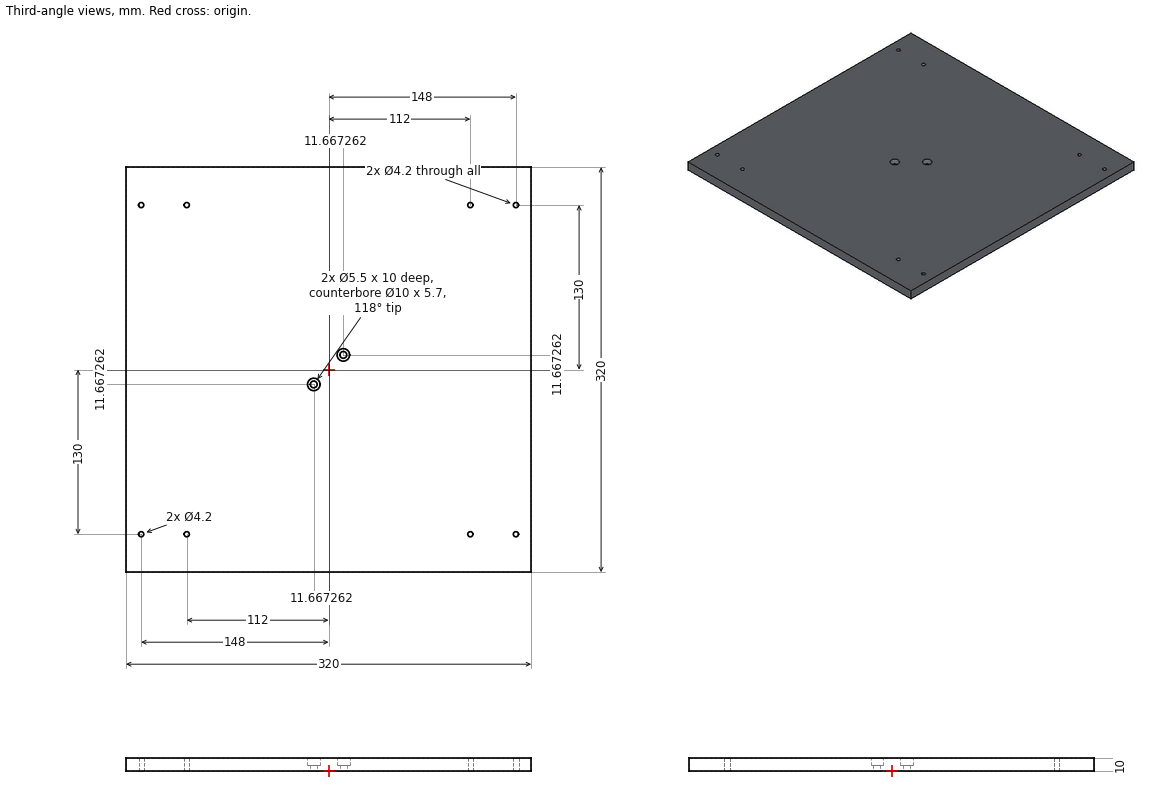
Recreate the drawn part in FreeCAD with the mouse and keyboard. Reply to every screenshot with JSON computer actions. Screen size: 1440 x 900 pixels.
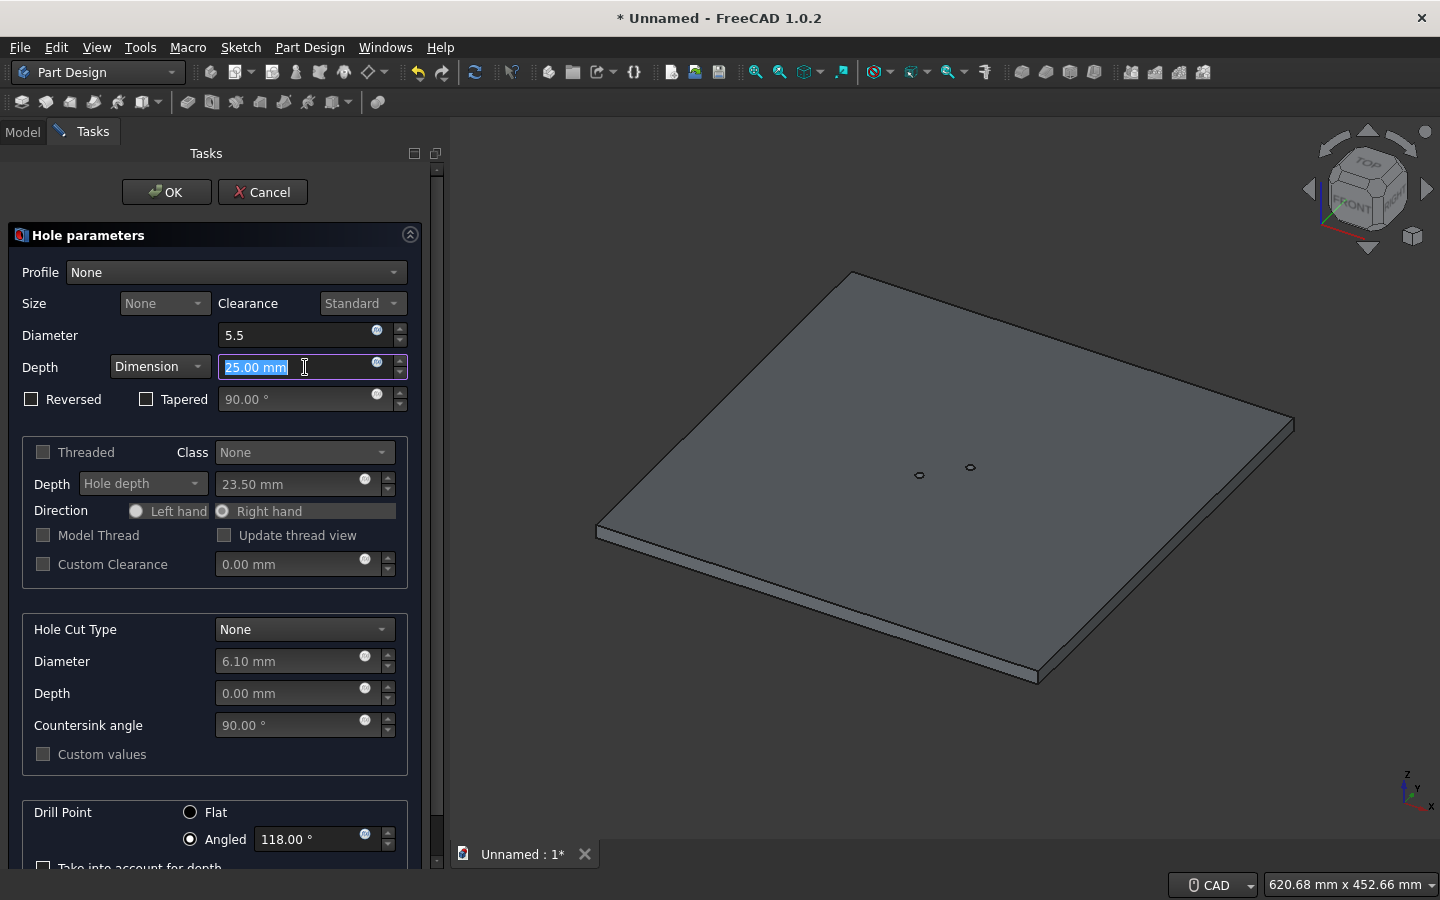
{"action": "type", "text": "10"}
{"action": "key", "text": "Tab"}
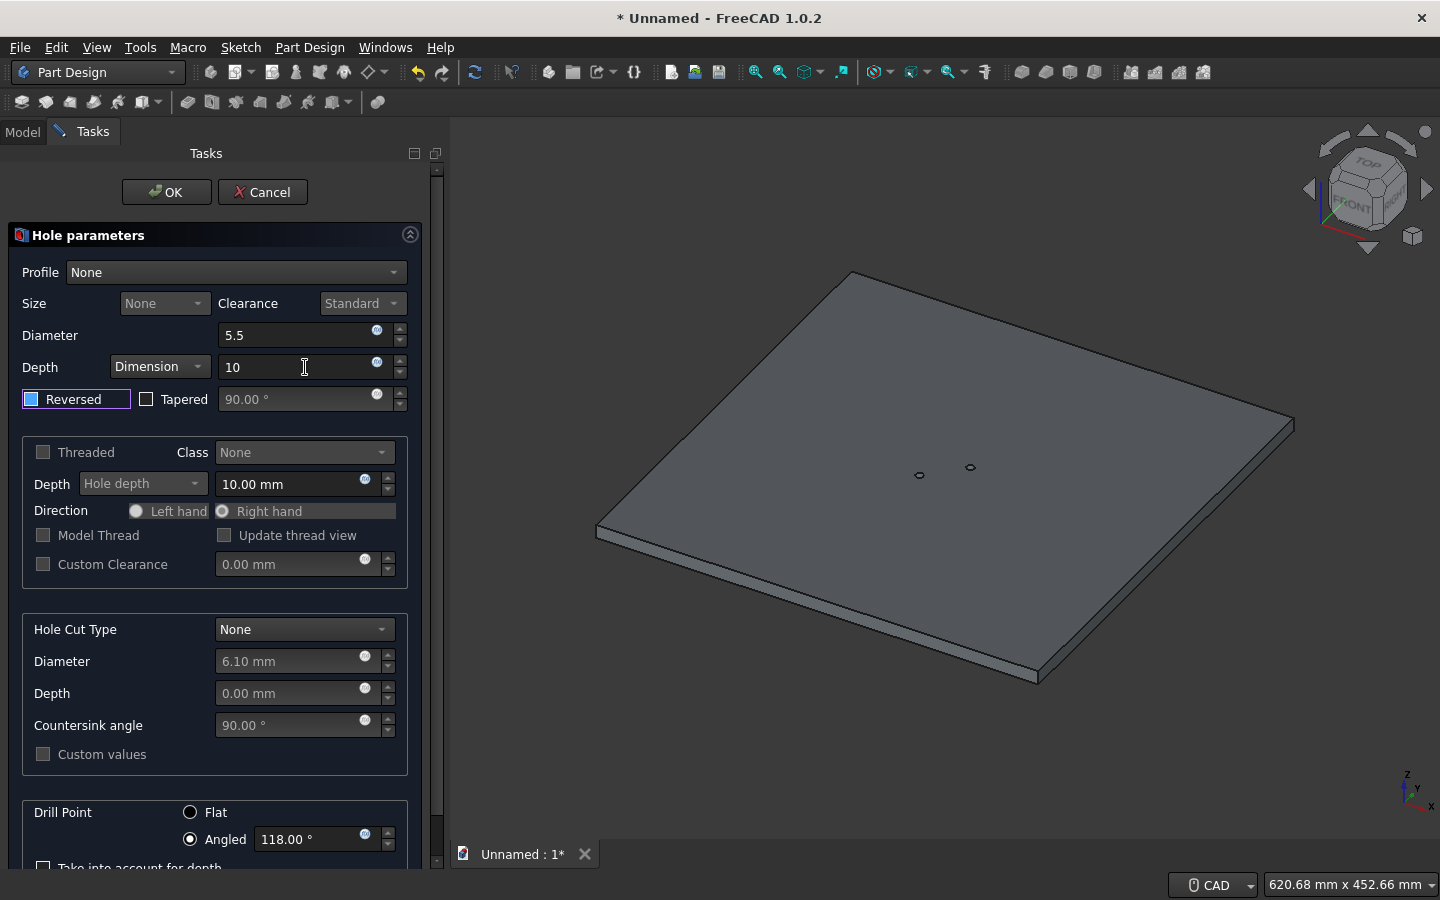
{"action": "left_click", "coordinate": [306, 630]}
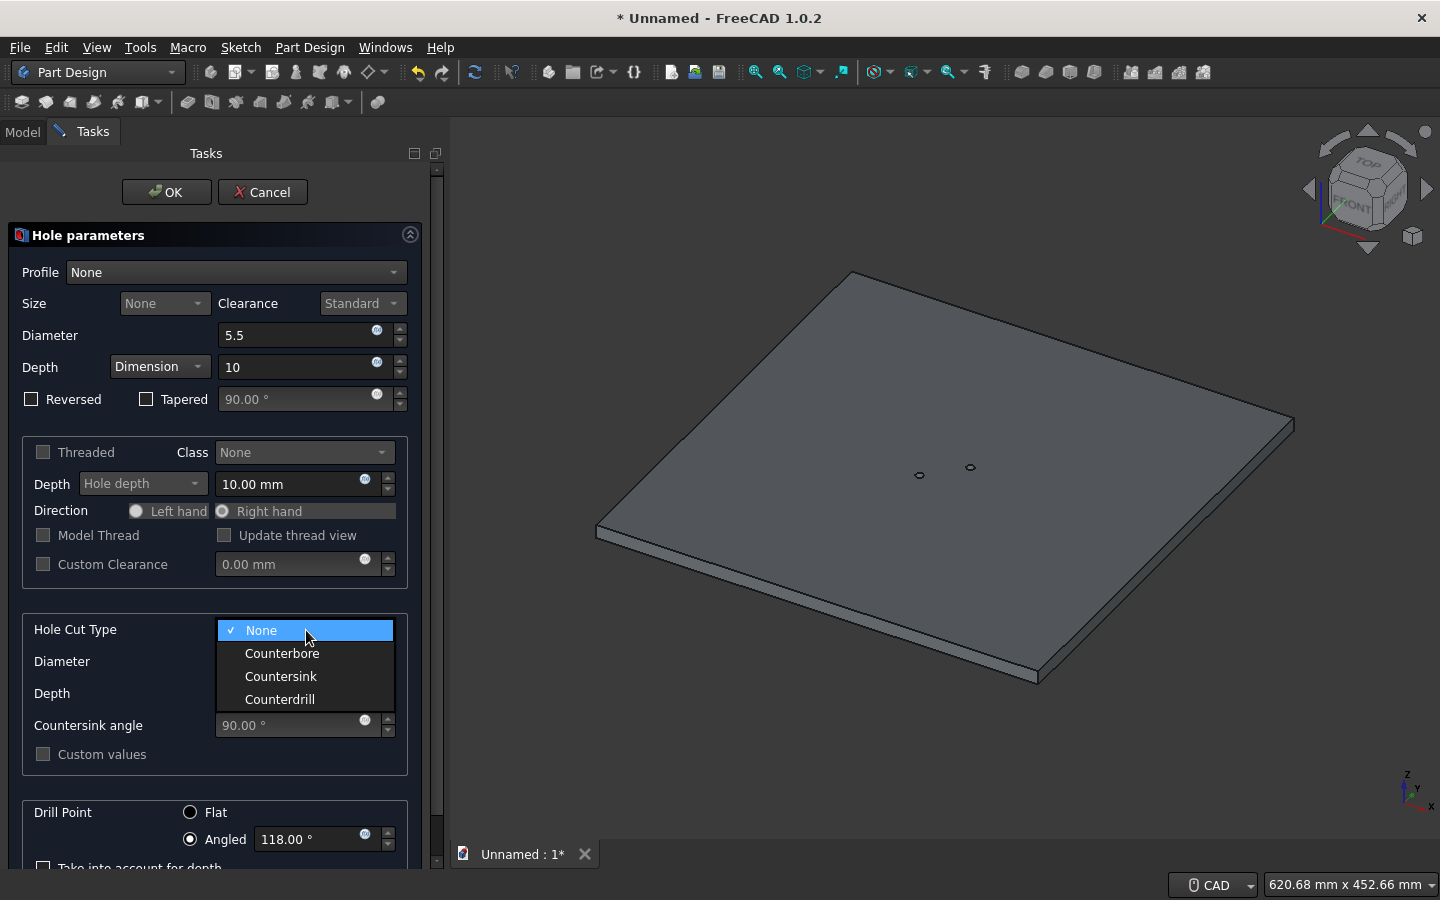
{"action": "left_click", "coordinate": [304, 654]}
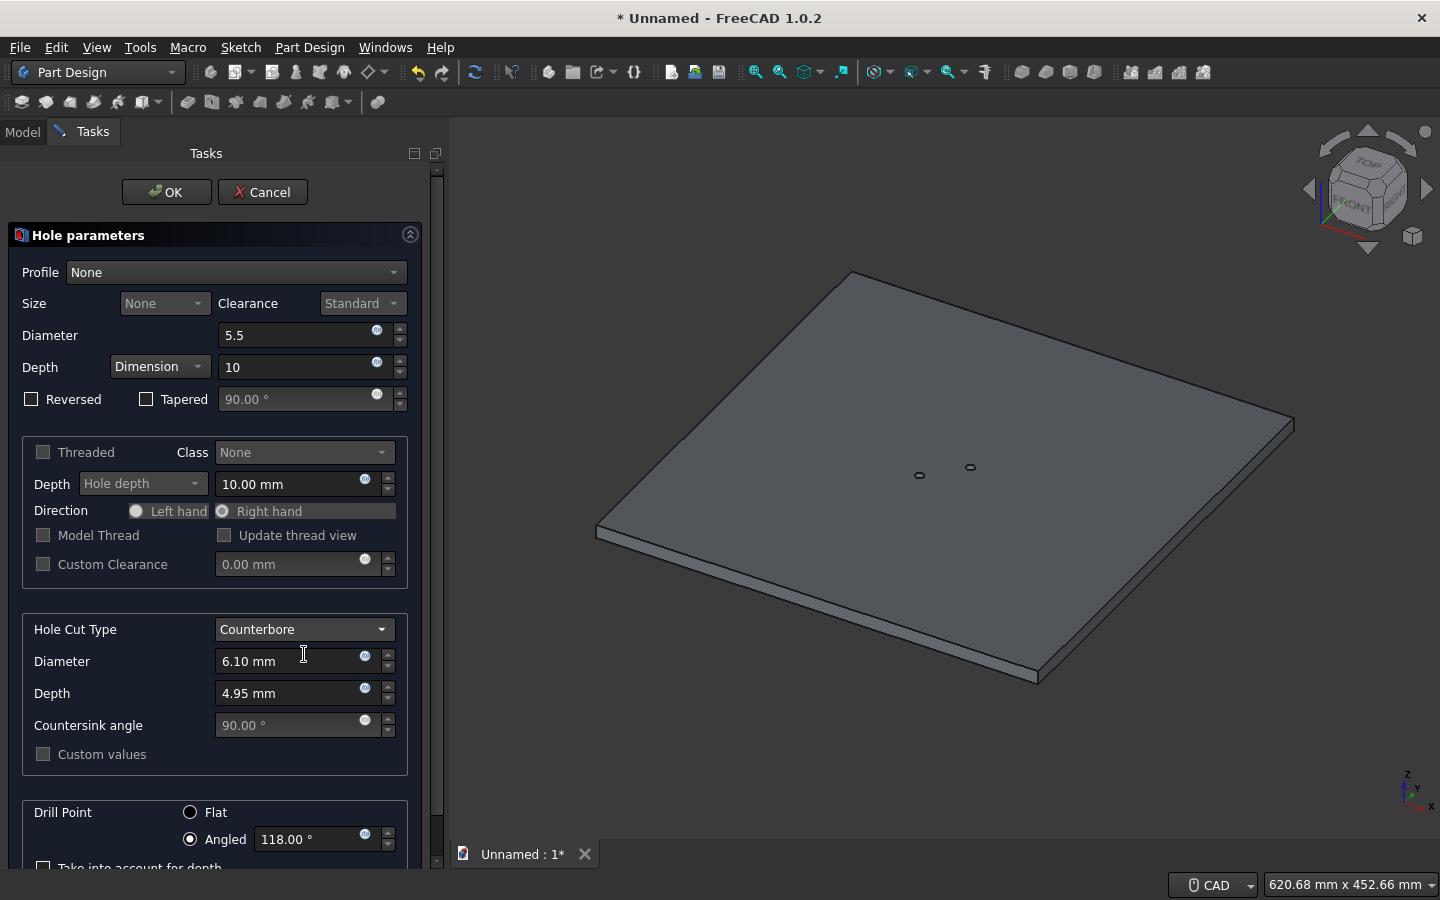
{"action": "triple_click", "coordinate": [298, 661]}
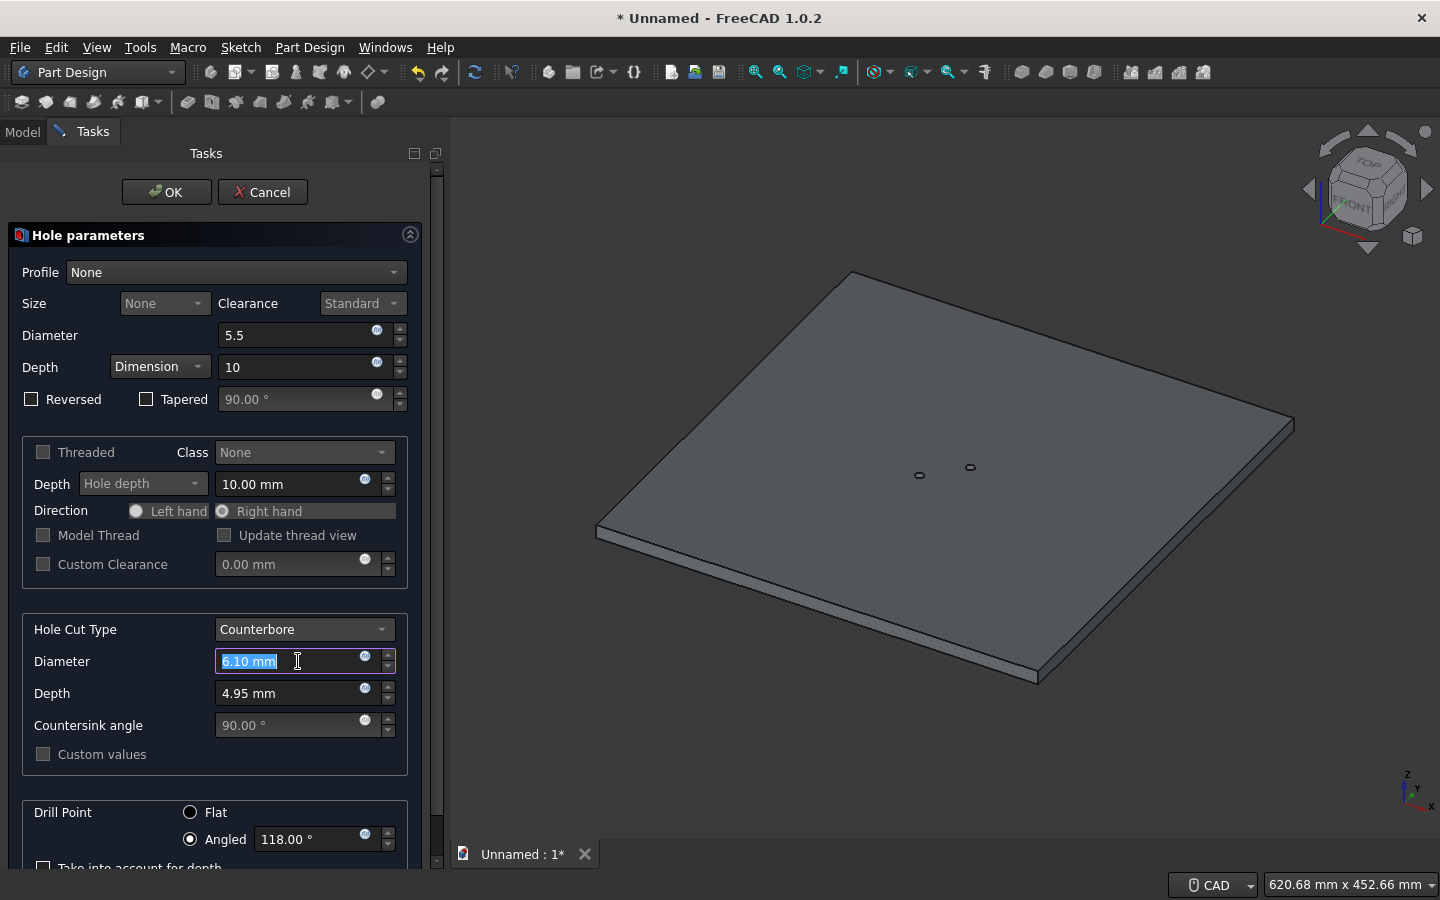
{"action": "type", "text": "10"}
{"action": "key", "text": "Tab"}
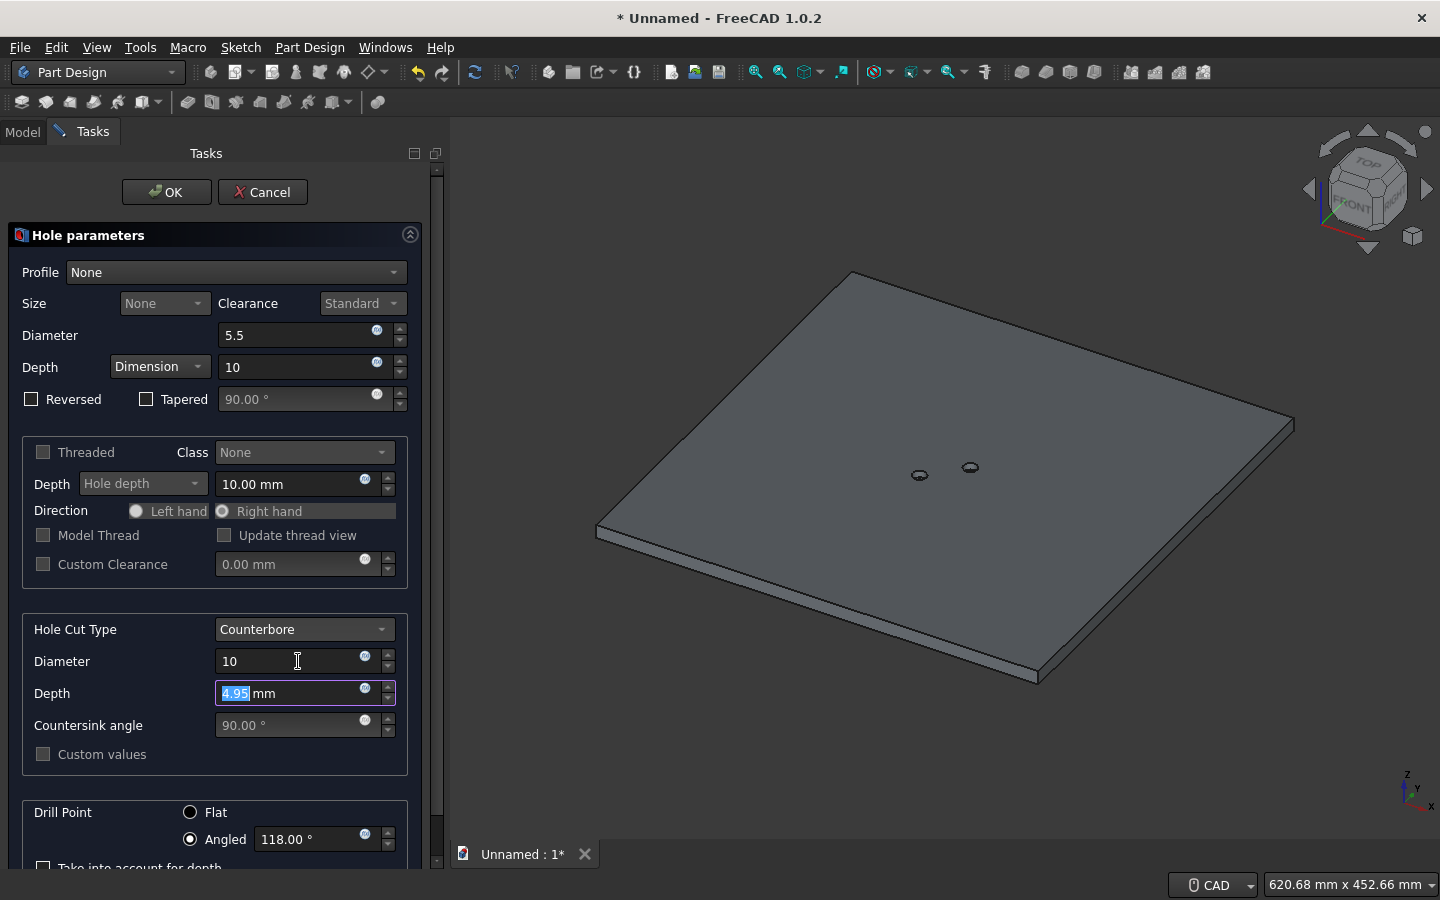
{"action": "type", "text": "5.7"}
{"action": "key", "text": "Tab"}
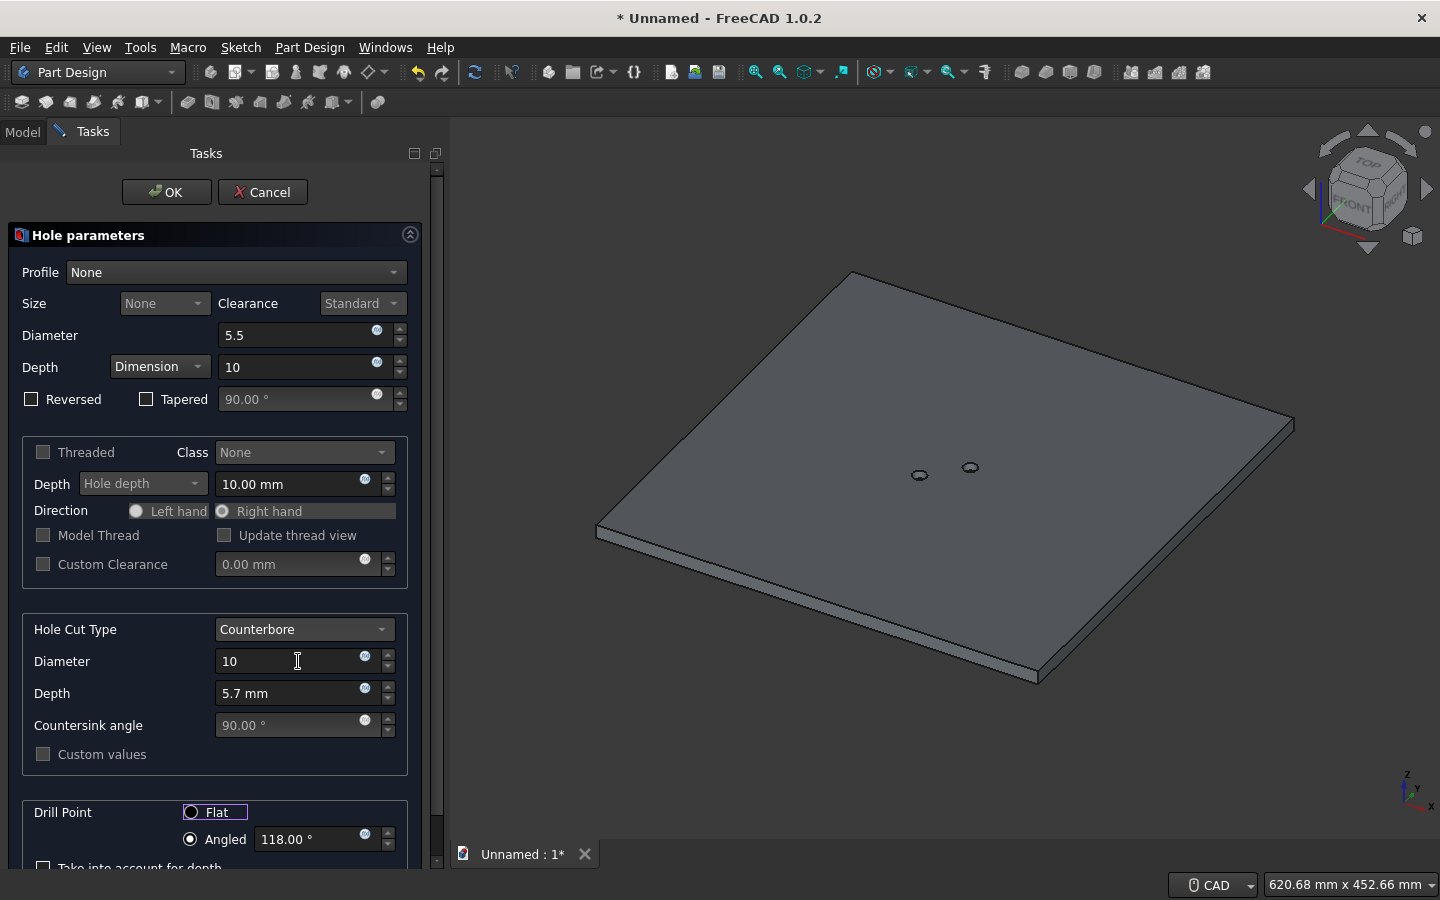
{"action": "left_click", "coordinate": [167, 192]}